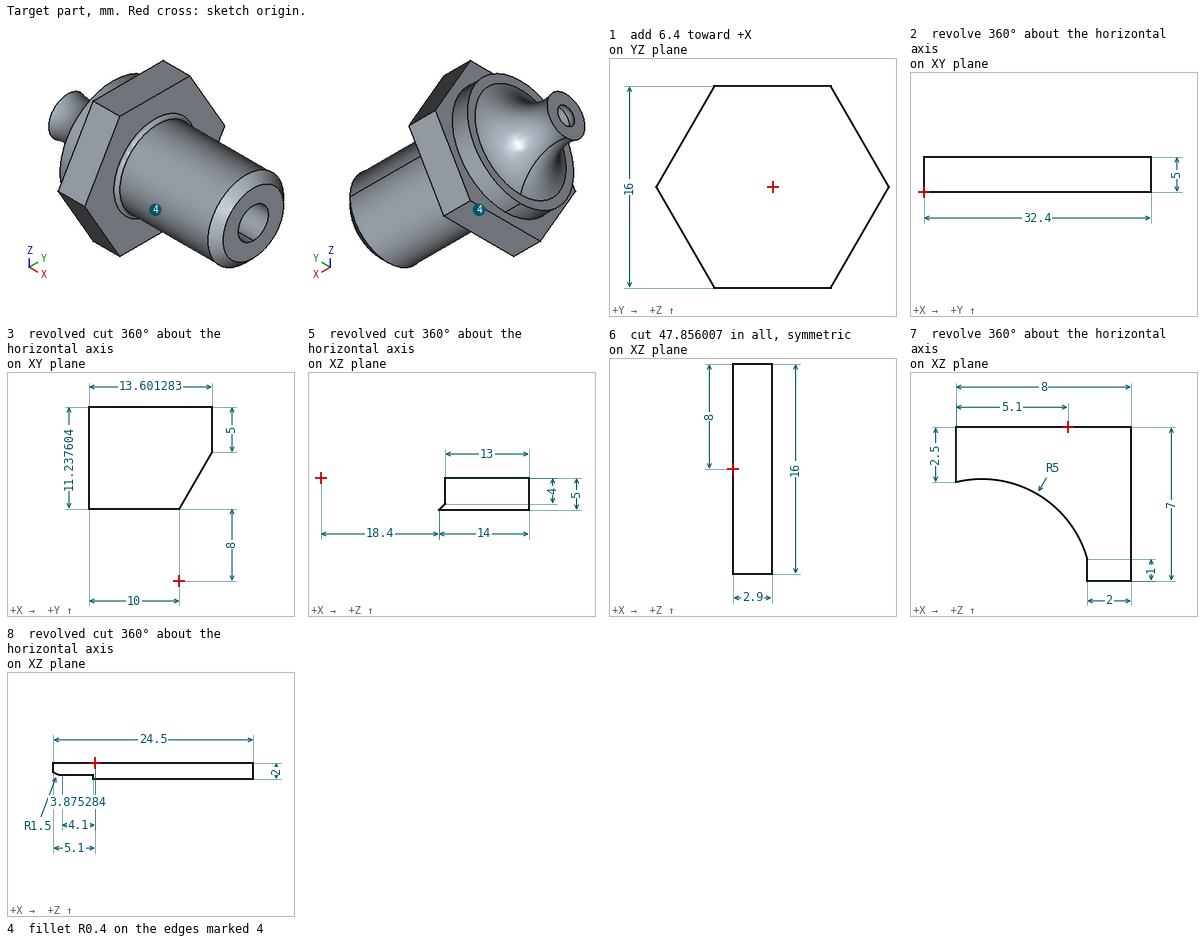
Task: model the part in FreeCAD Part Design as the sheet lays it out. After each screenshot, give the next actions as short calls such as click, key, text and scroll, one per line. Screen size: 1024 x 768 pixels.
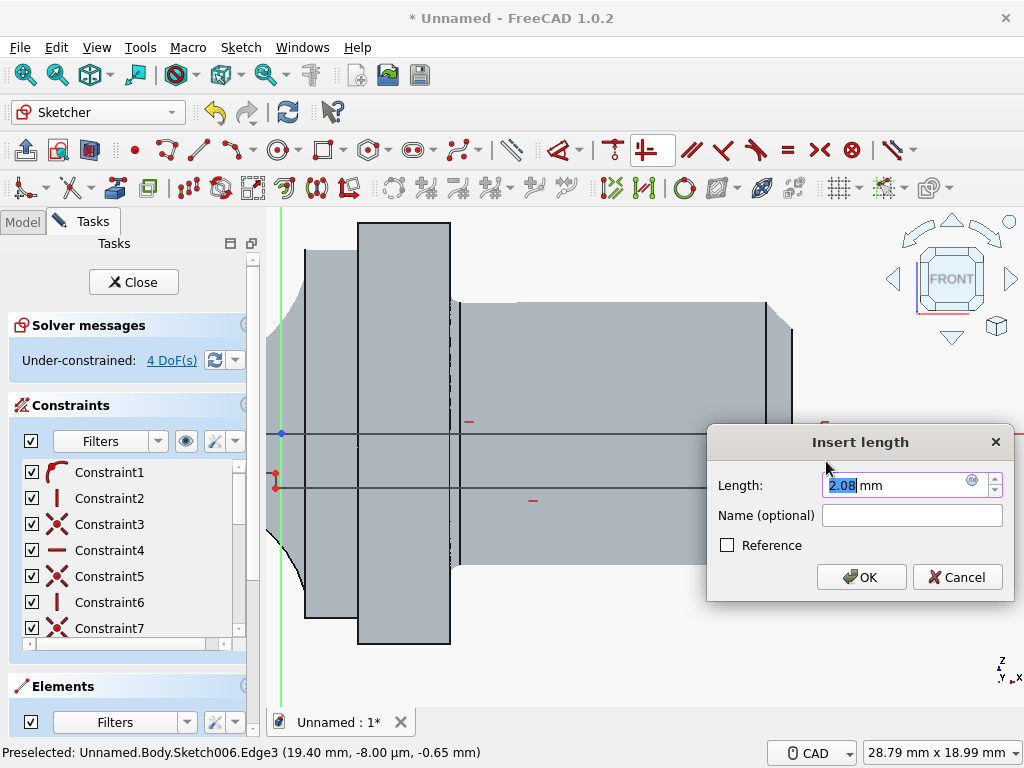
text(2)
key(Return)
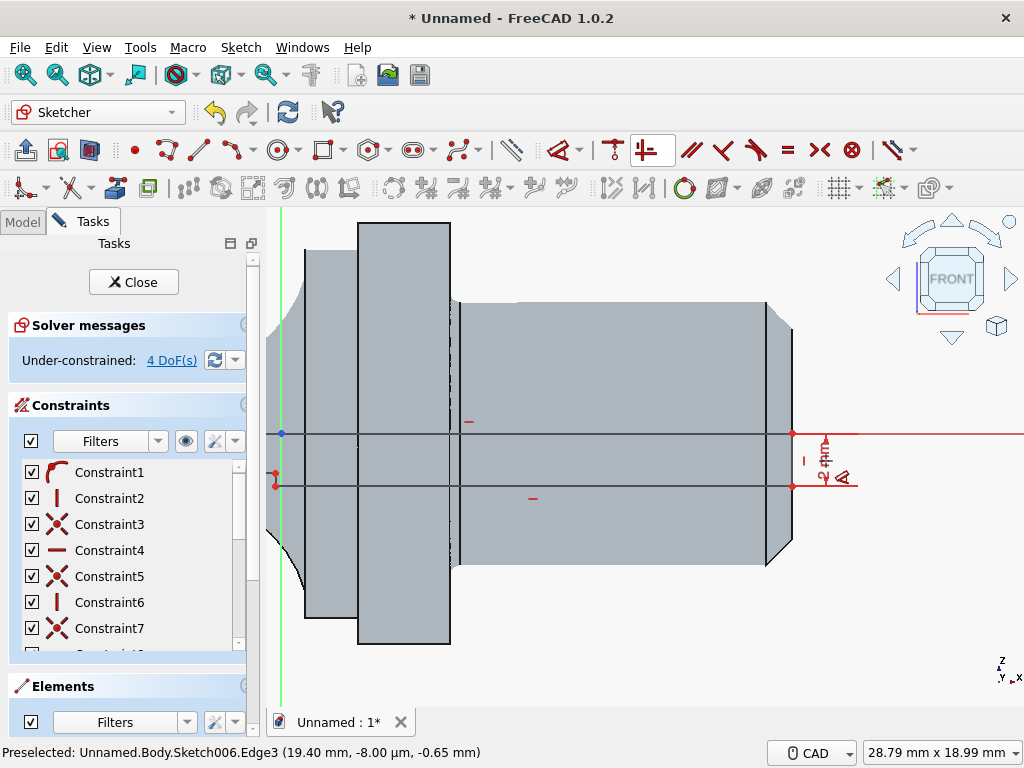
click(341, 434)
click(543, 400)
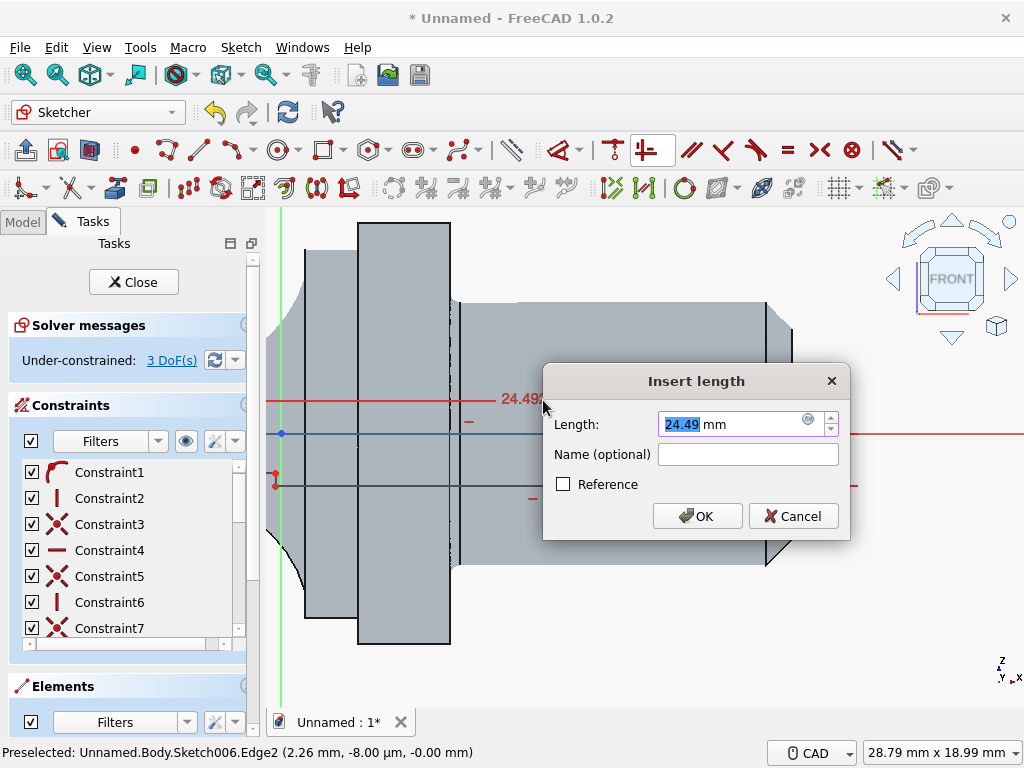
text(24.5)
key(Return)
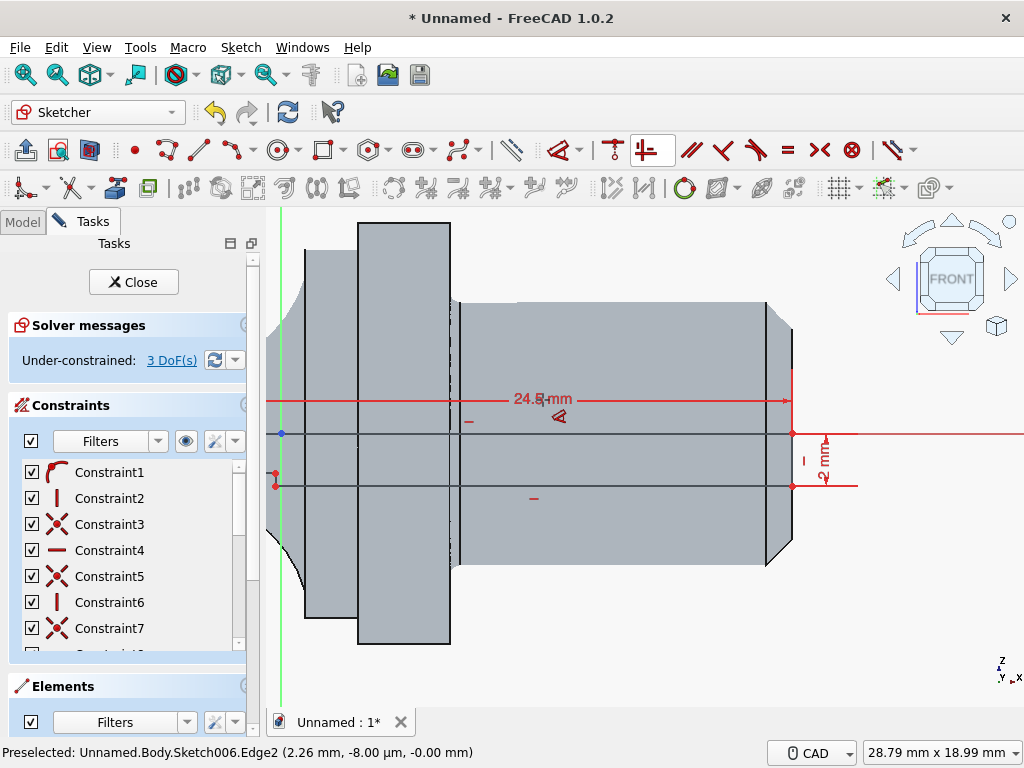
scroll(794, 451, down, 2)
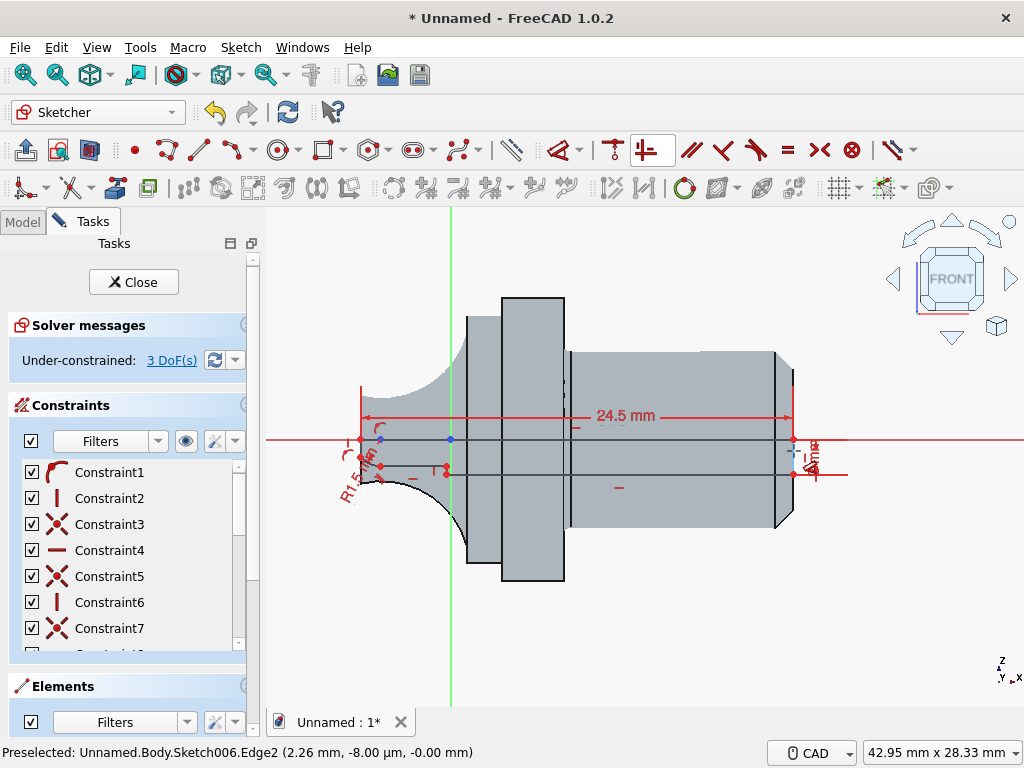
click(361, 458)
click(406, 406)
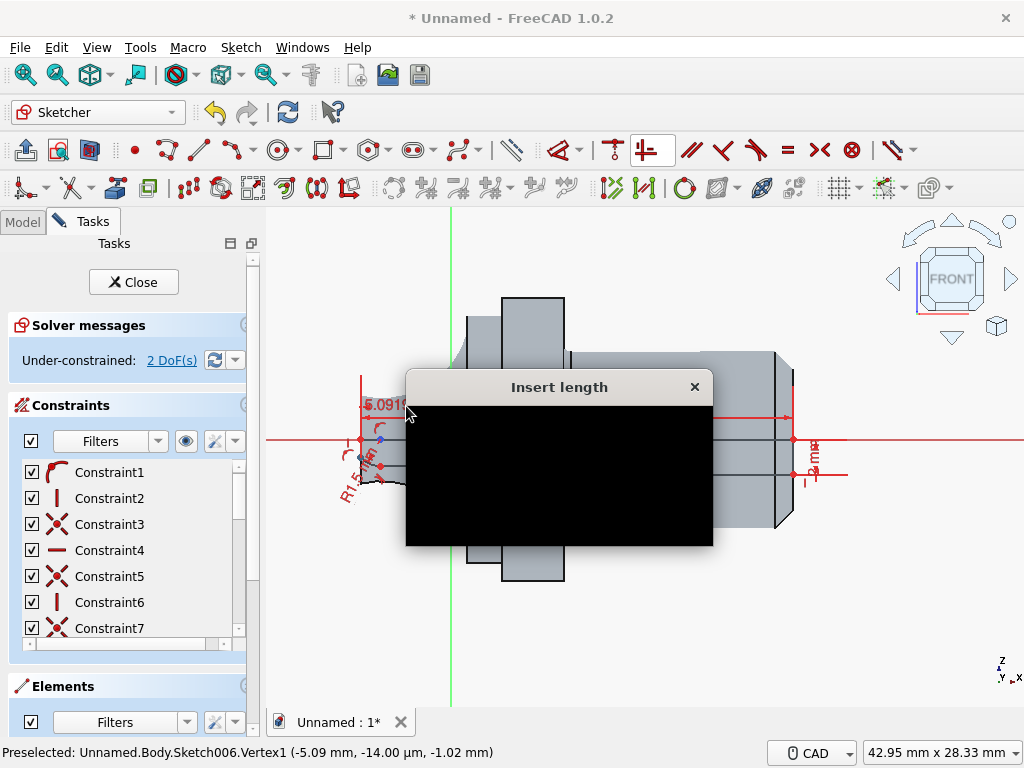
text(5.1)
key(Return)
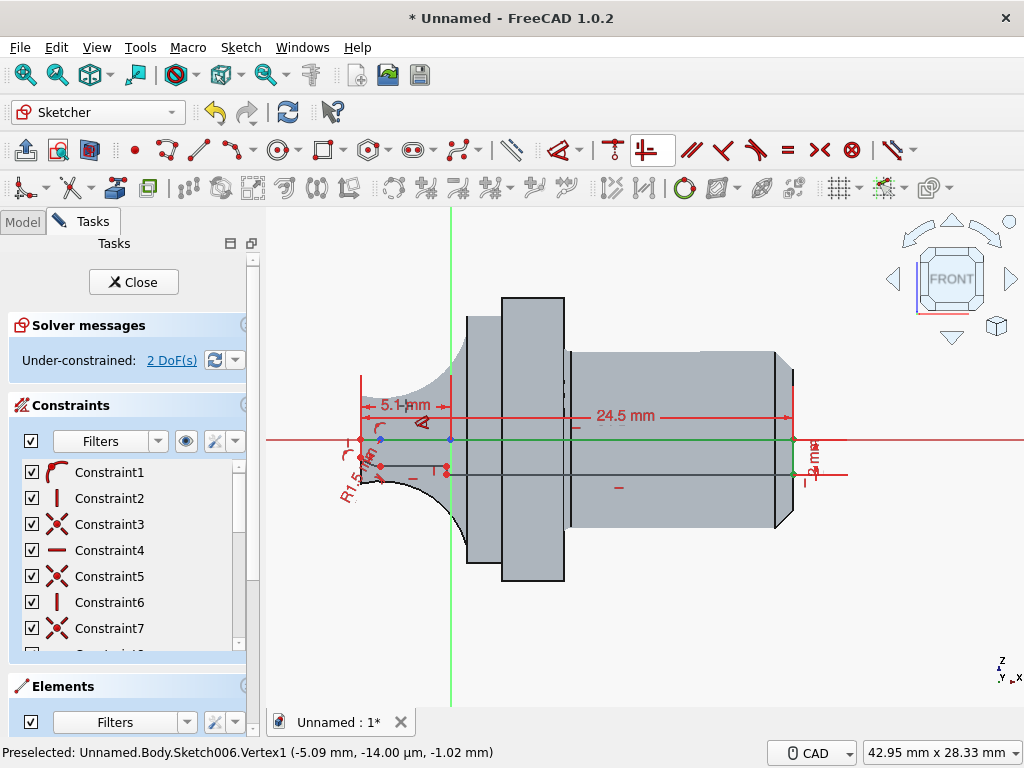
click(380, 466)
click(415, 500)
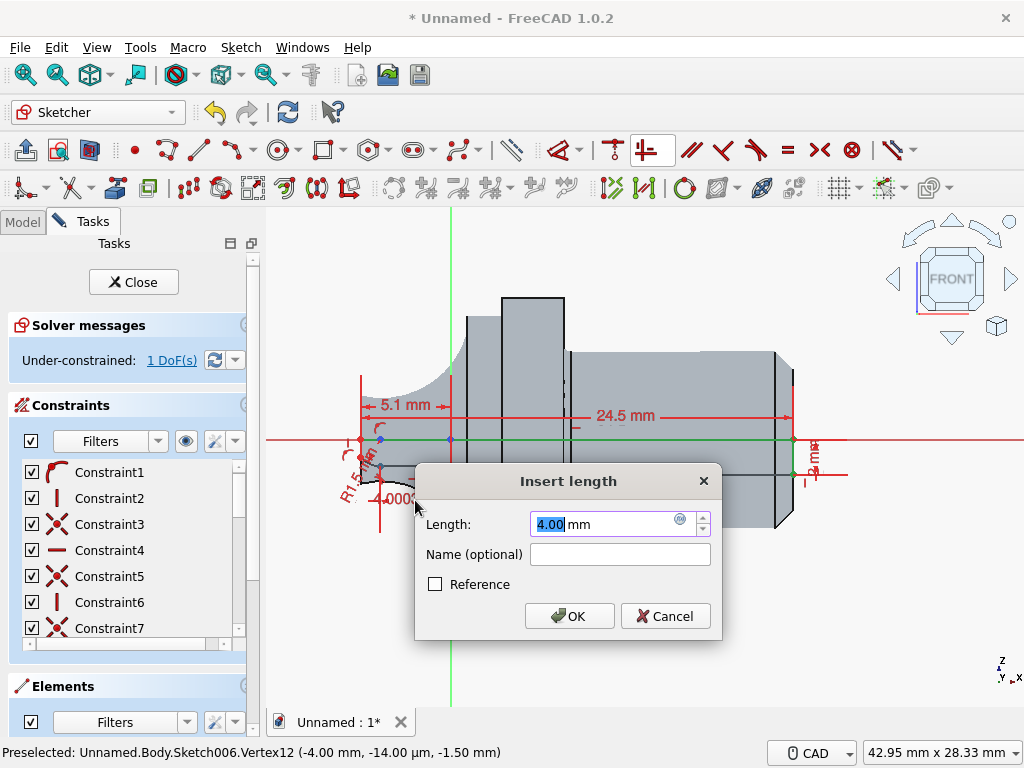
text(4.1)
key(Return)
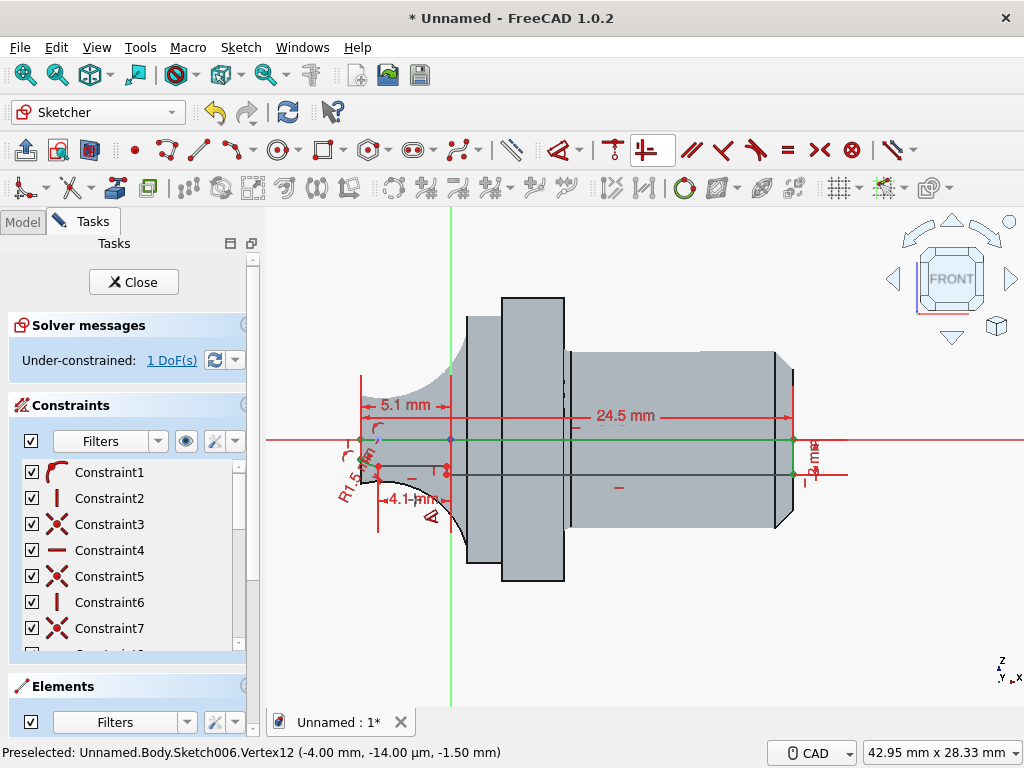
click(426, 466)
click(413, 524)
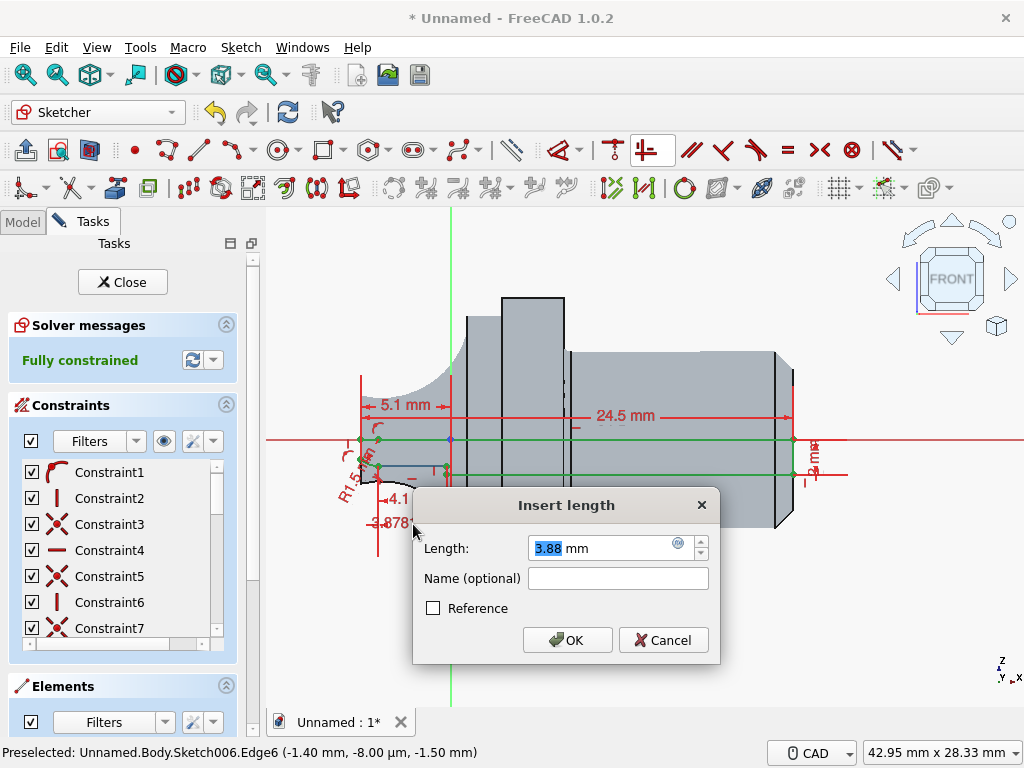
text(3.875284)
key(Return)
key(Escape)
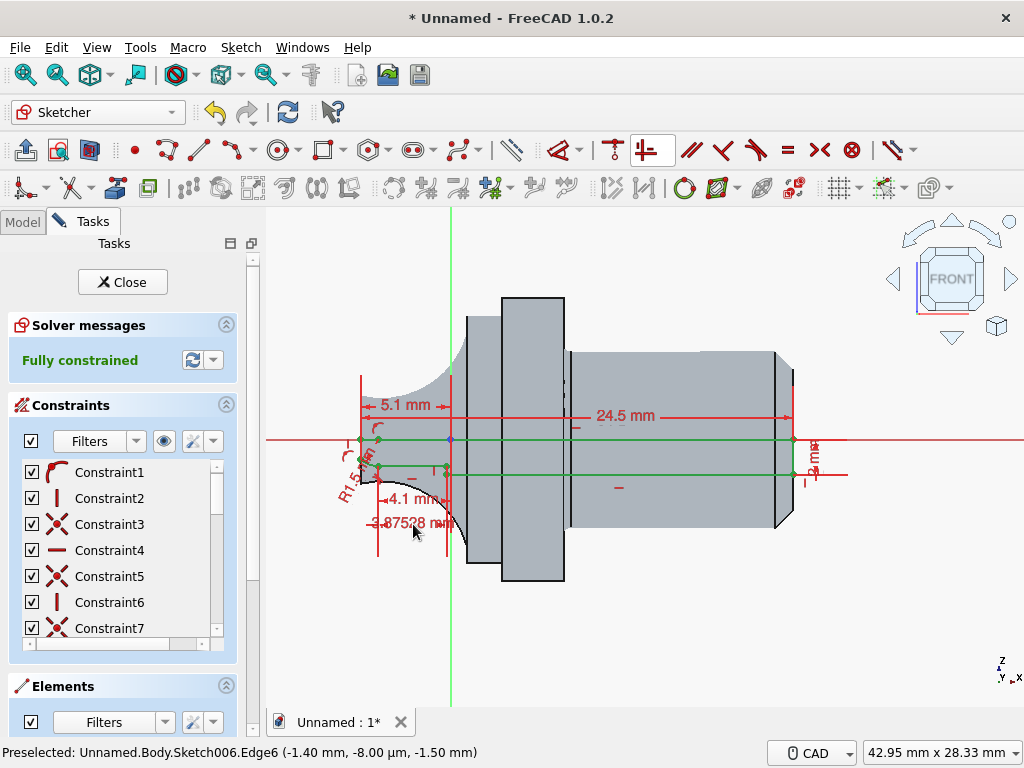
click(123, 282)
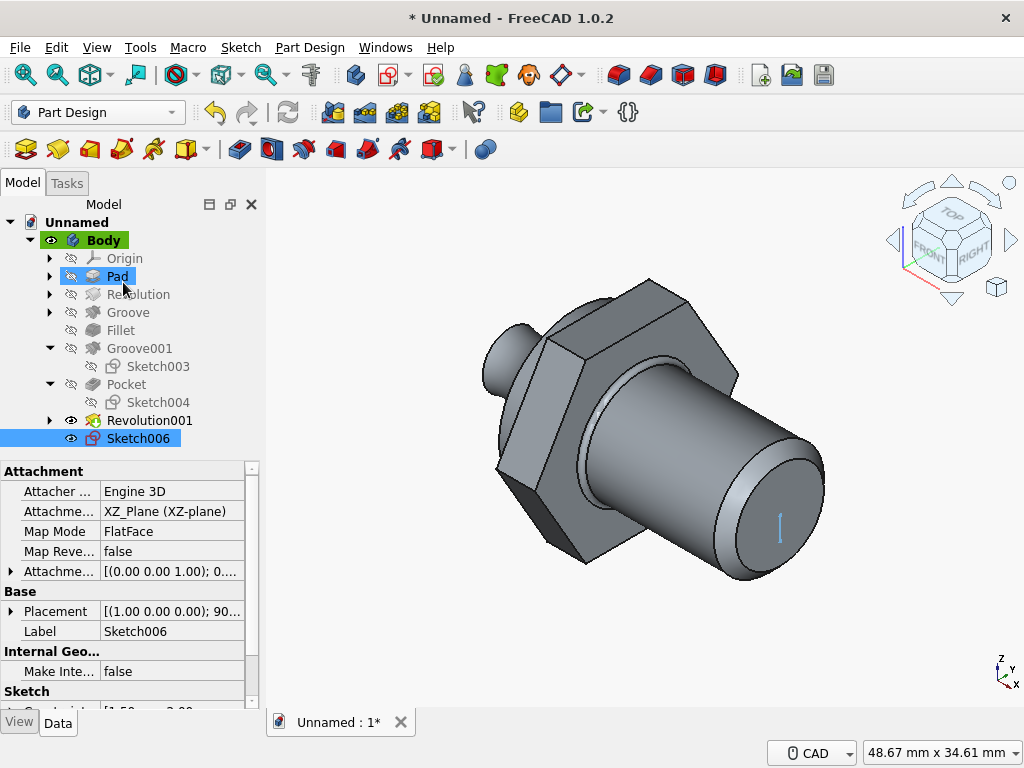
click(304, 150)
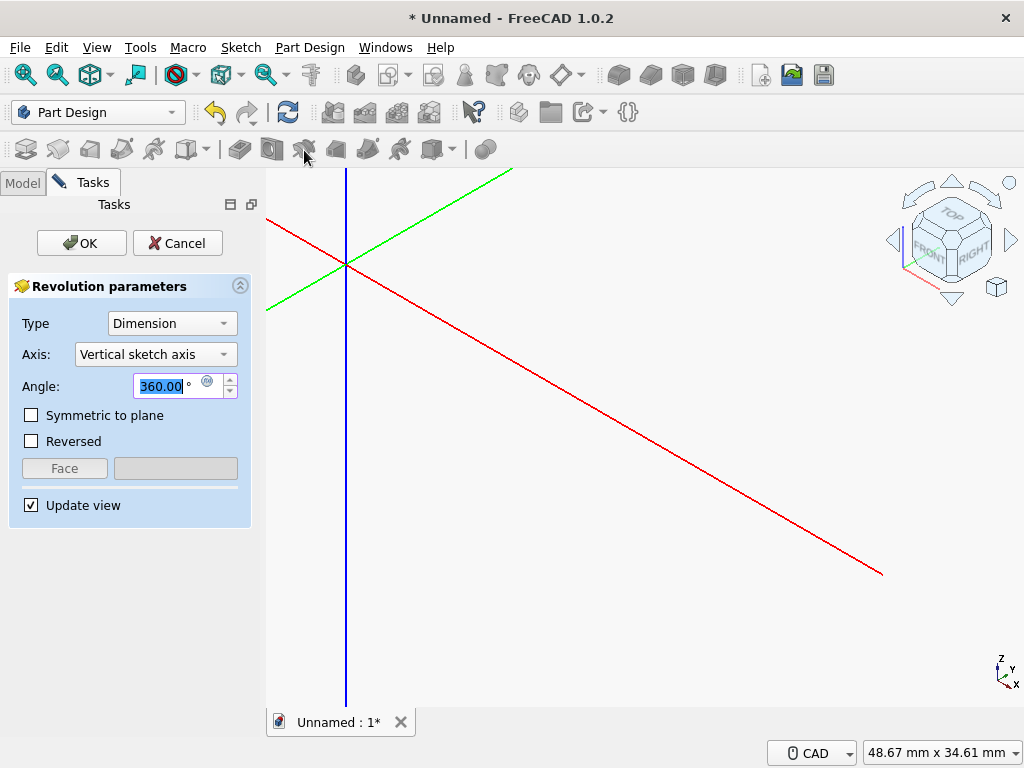
click(156, 354)